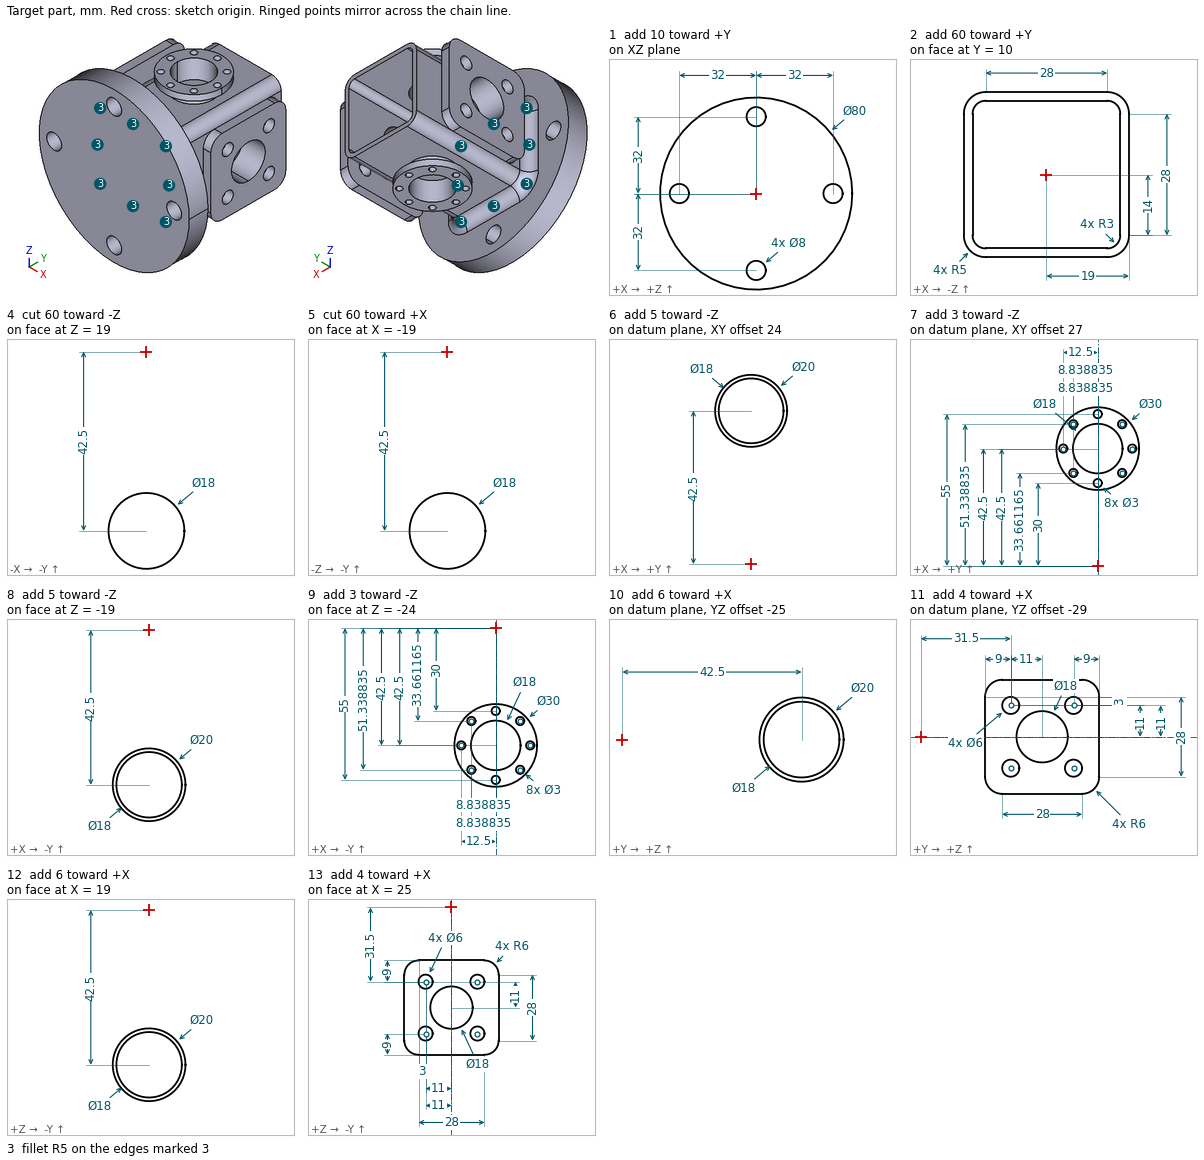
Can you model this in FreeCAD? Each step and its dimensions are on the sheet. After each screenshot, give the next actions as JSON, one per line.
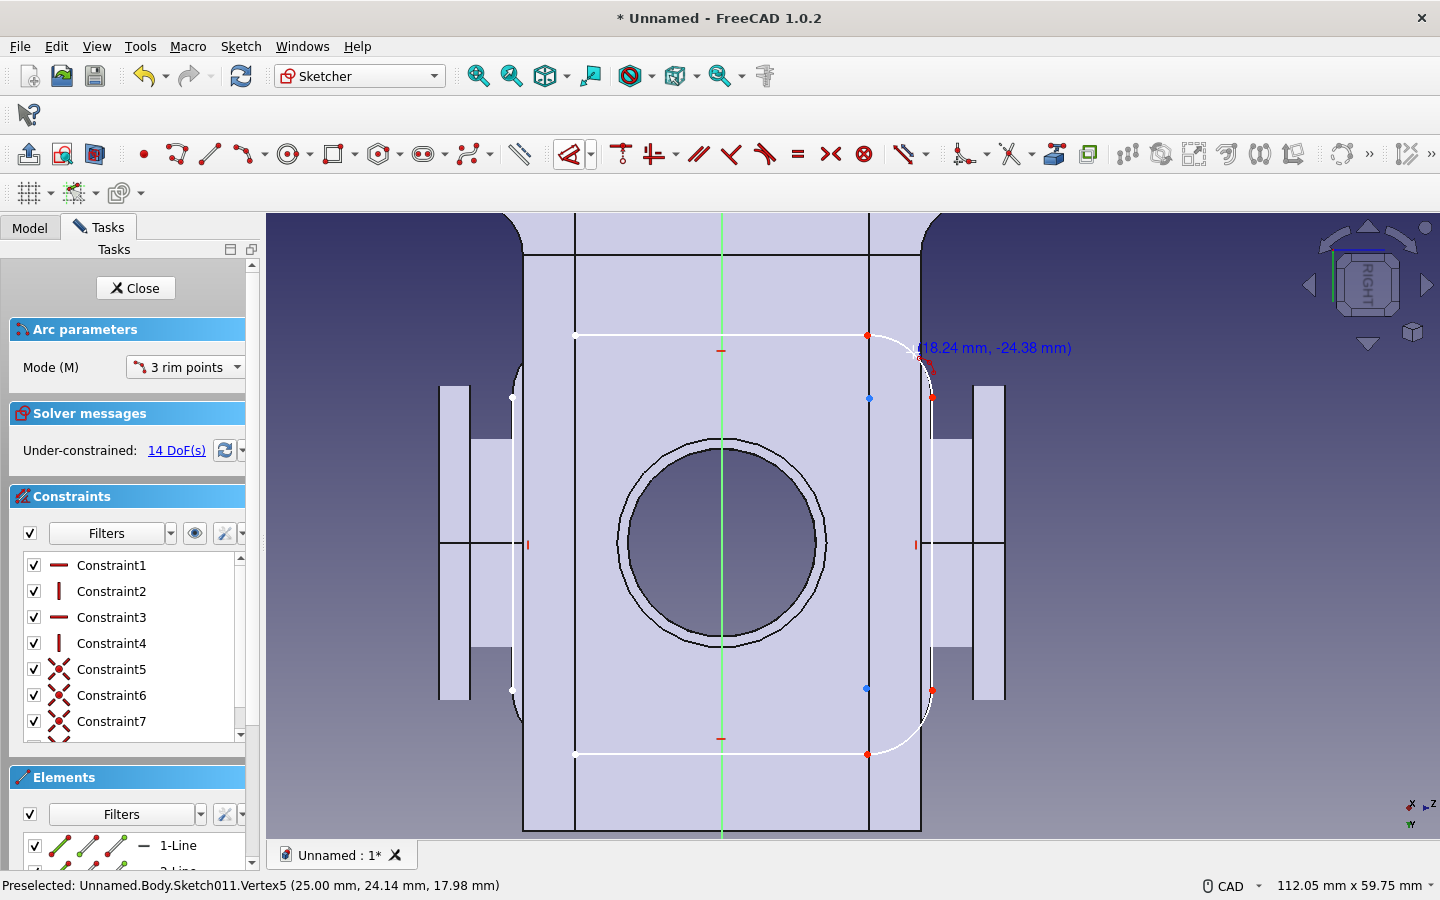
{"action": "left_click", "coordinate": [576, 335]}
{"action": "left_click", "coordinate": [513, 398]}
{"action": "left_click", "coordinate": [531, 352]}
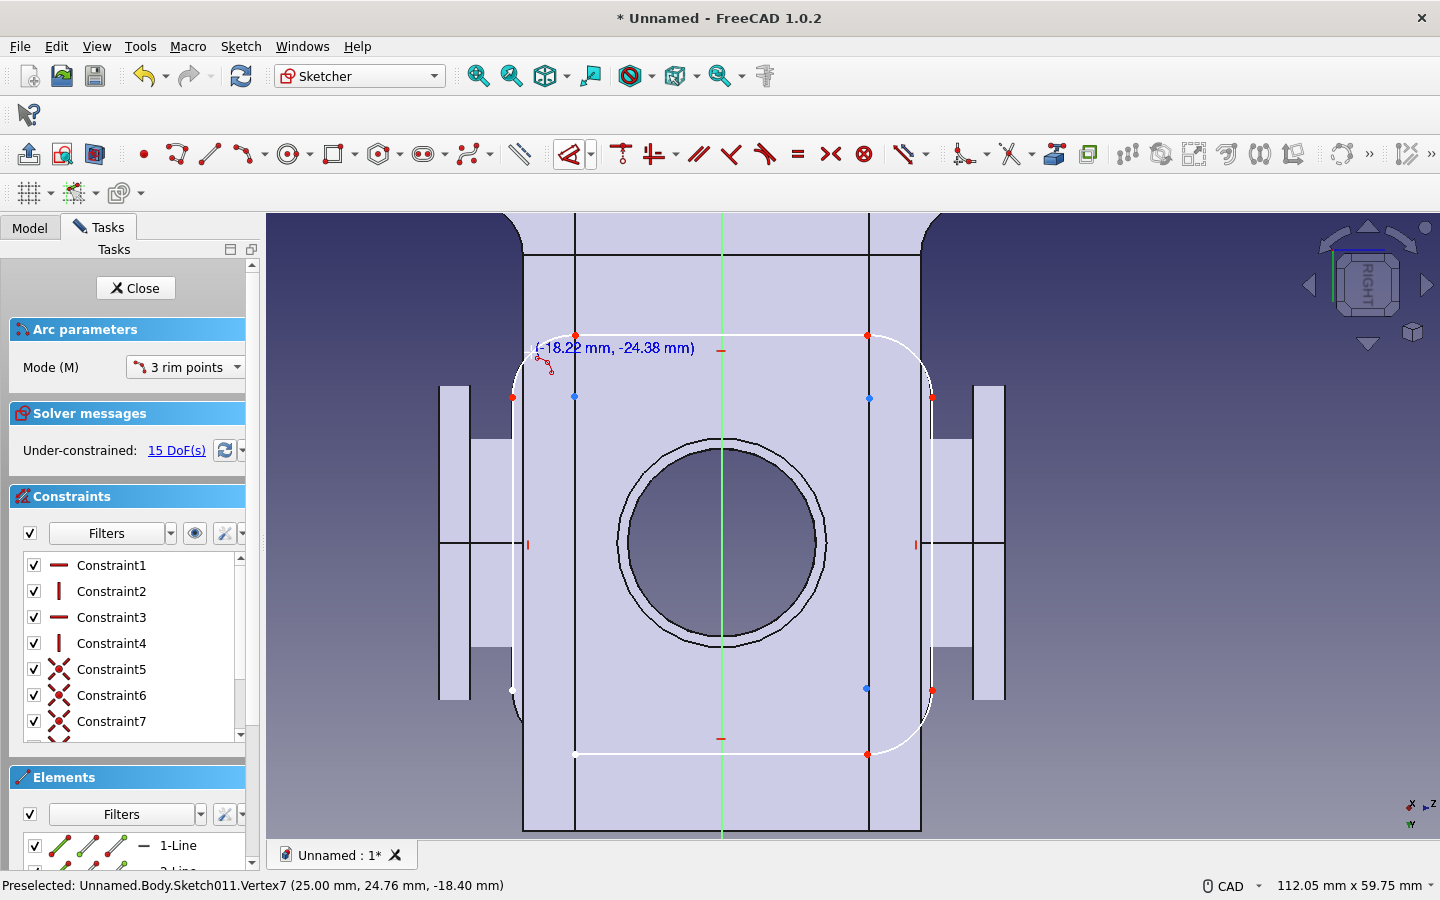
{"action": "left_click", "coordinate": [513, 690]}
{"action": "left_click", "coordinate": [576, 754]}
{"action": "left_click", "coordinate": [531, 734]}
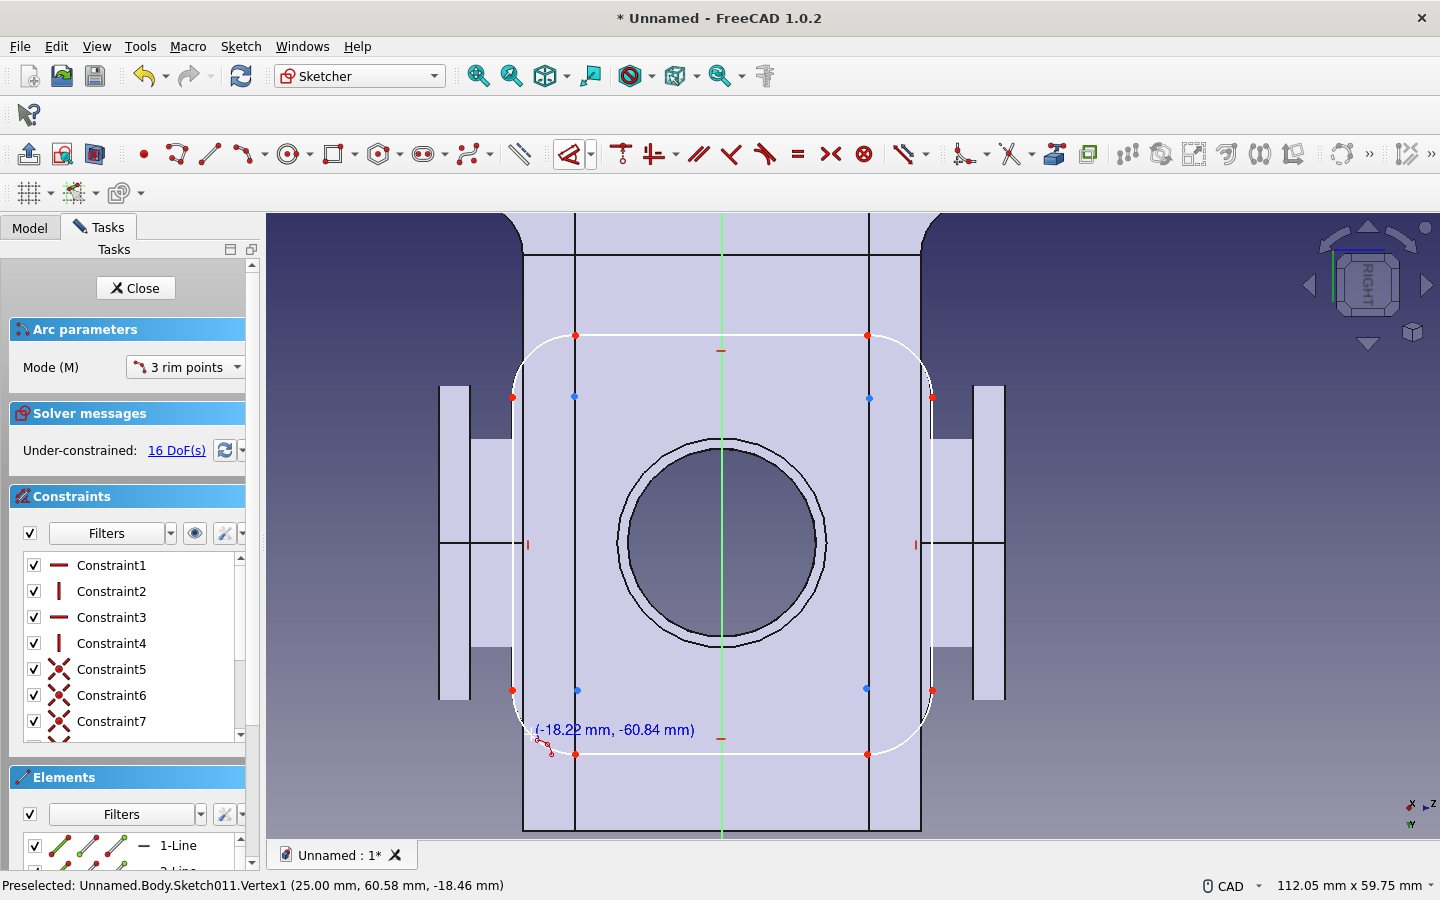
{"action": "key", "text": "g c"}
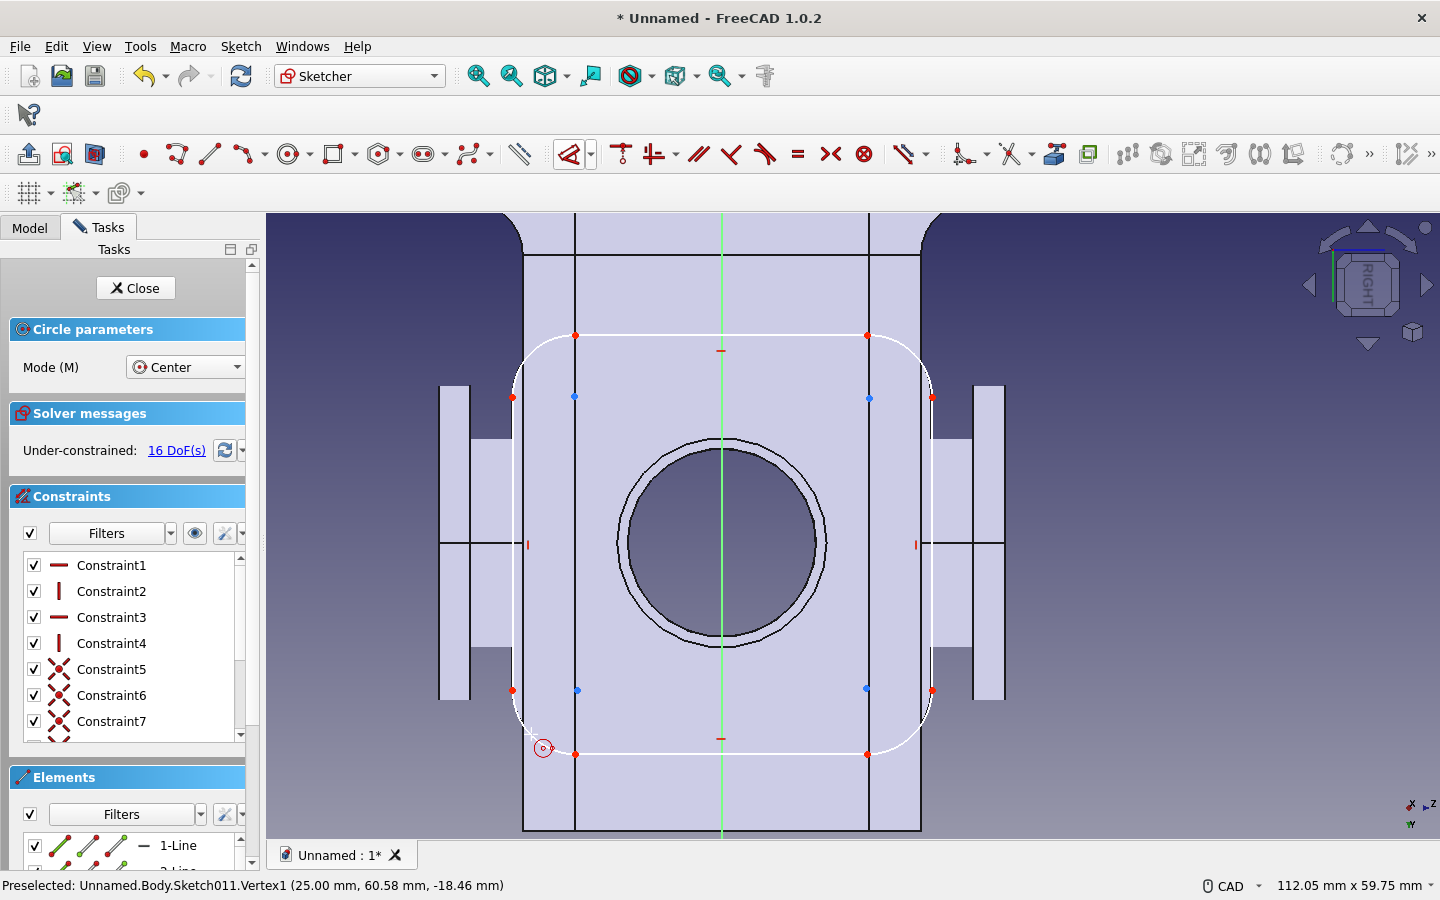
{"action": "left_click", "coordinate": [607, 428]}
{"action": "mouse_move", "coordinate": [629, 405]}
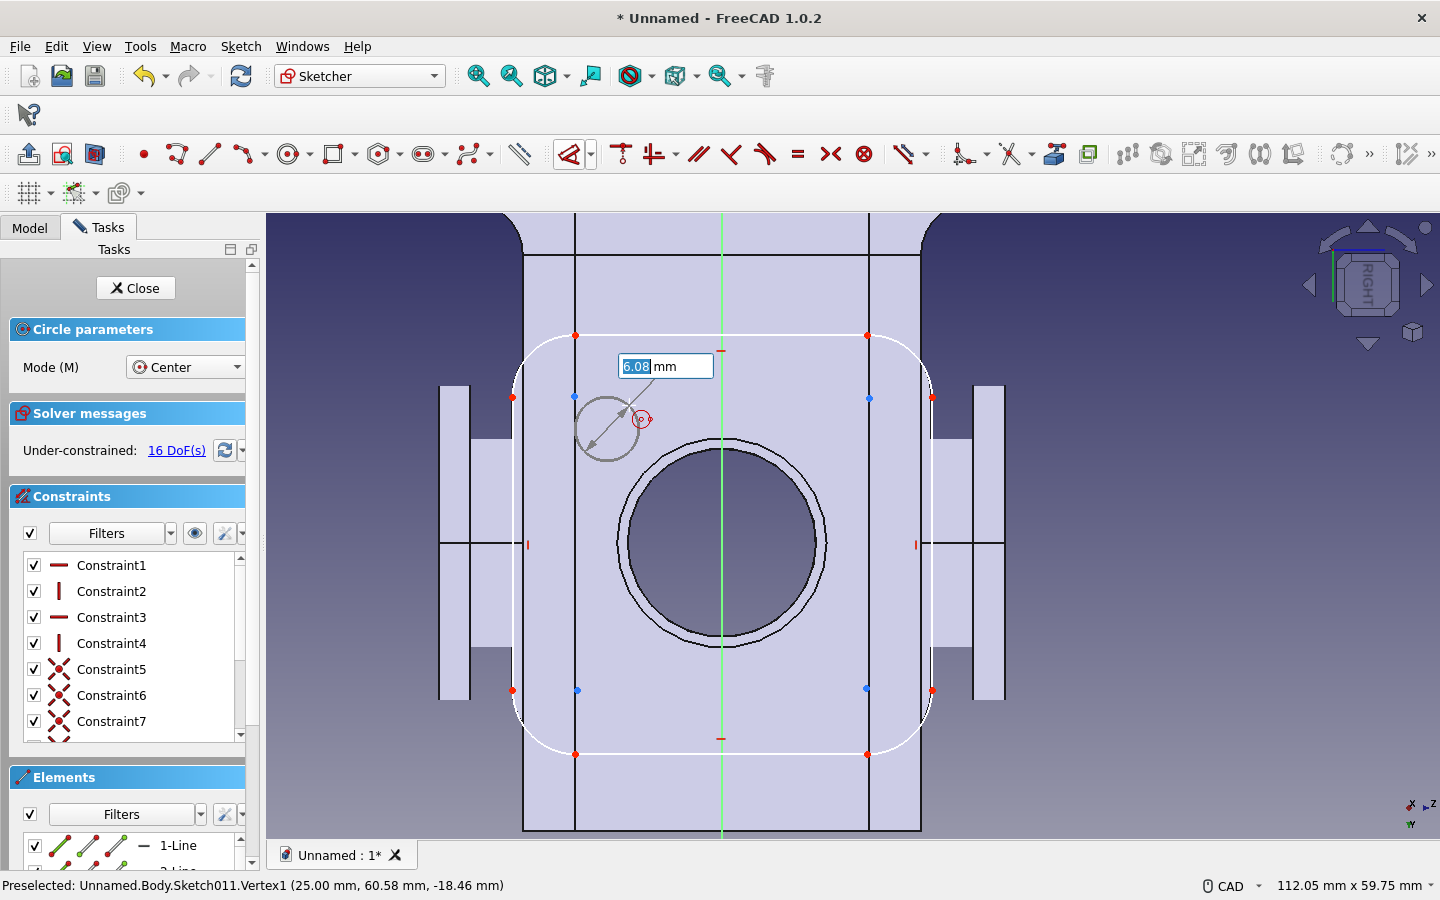
{"action": "type", "text": "6"}
{"action": "key", "text": "Return"}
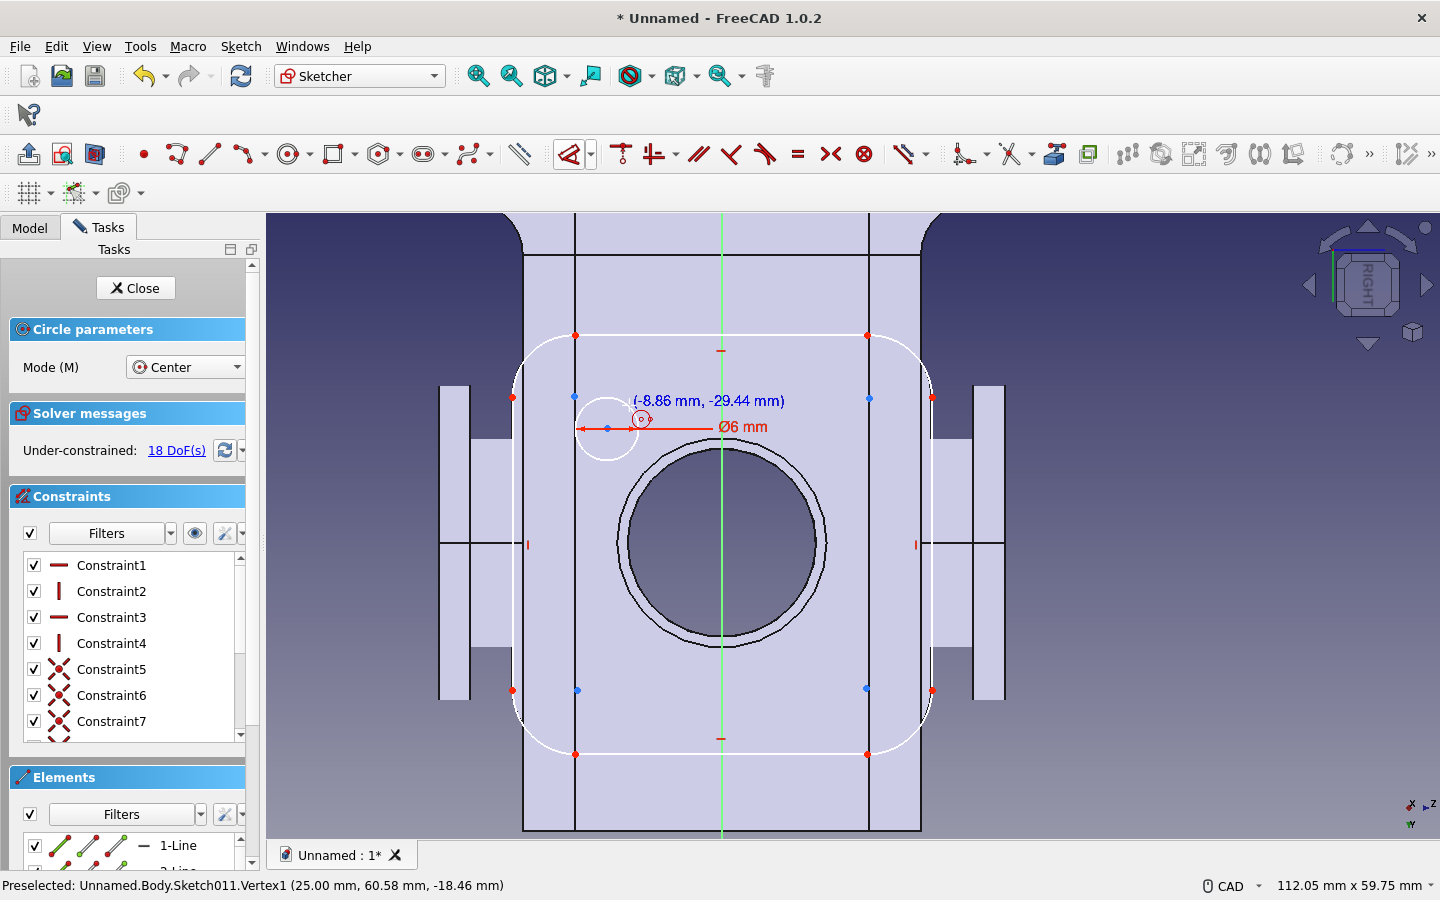
{"action": "left_click", "coordinate": [837, 428]}
{"action": "mouse_move", "coordinate": [815, 405]}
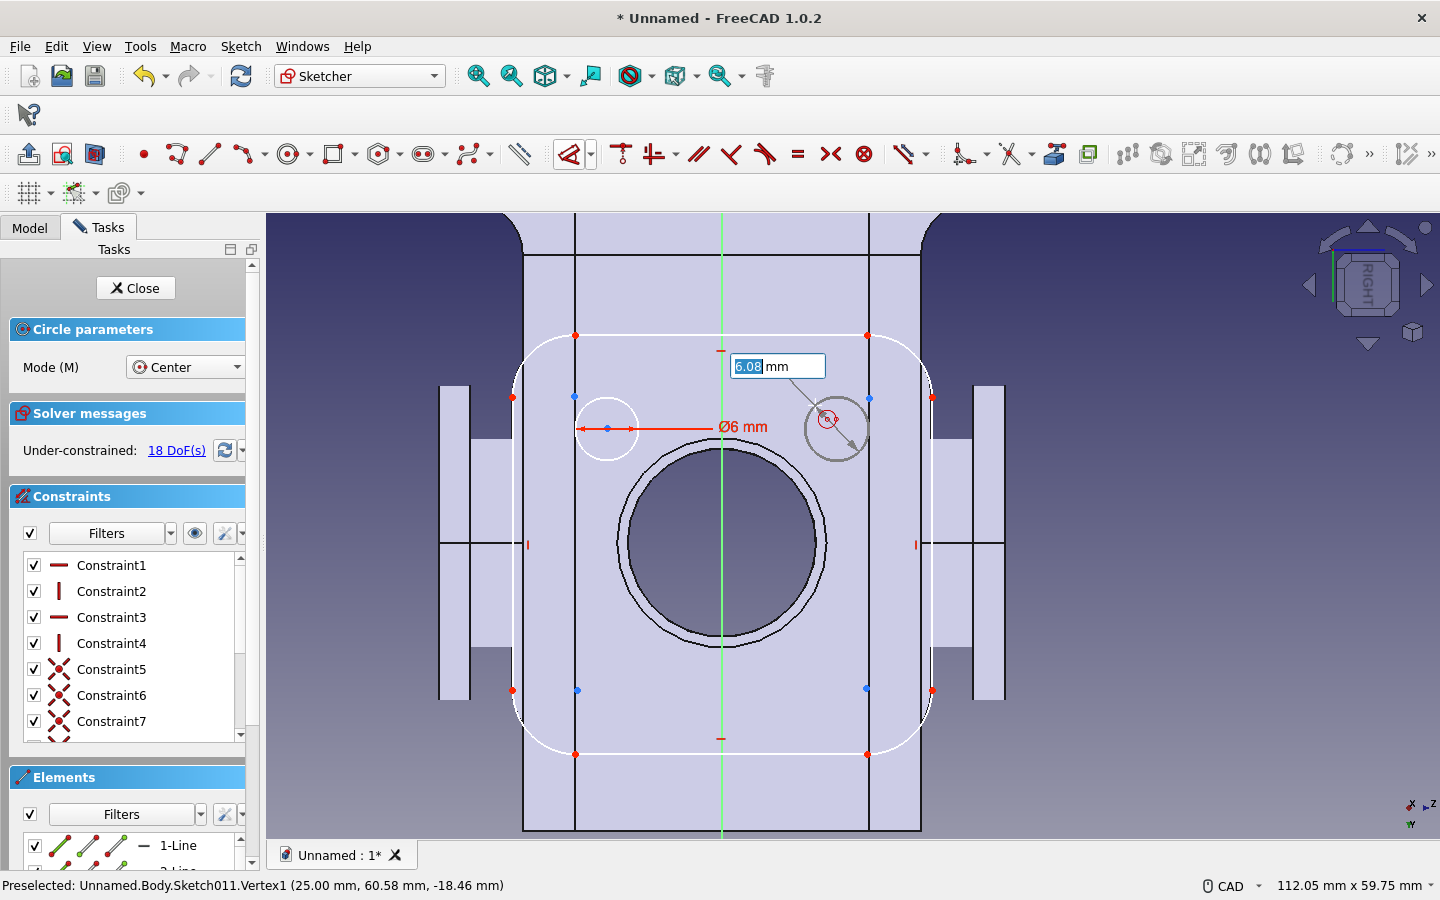
{"action": "type", "text": "6"}
{"action": "key", "text": "Return"}